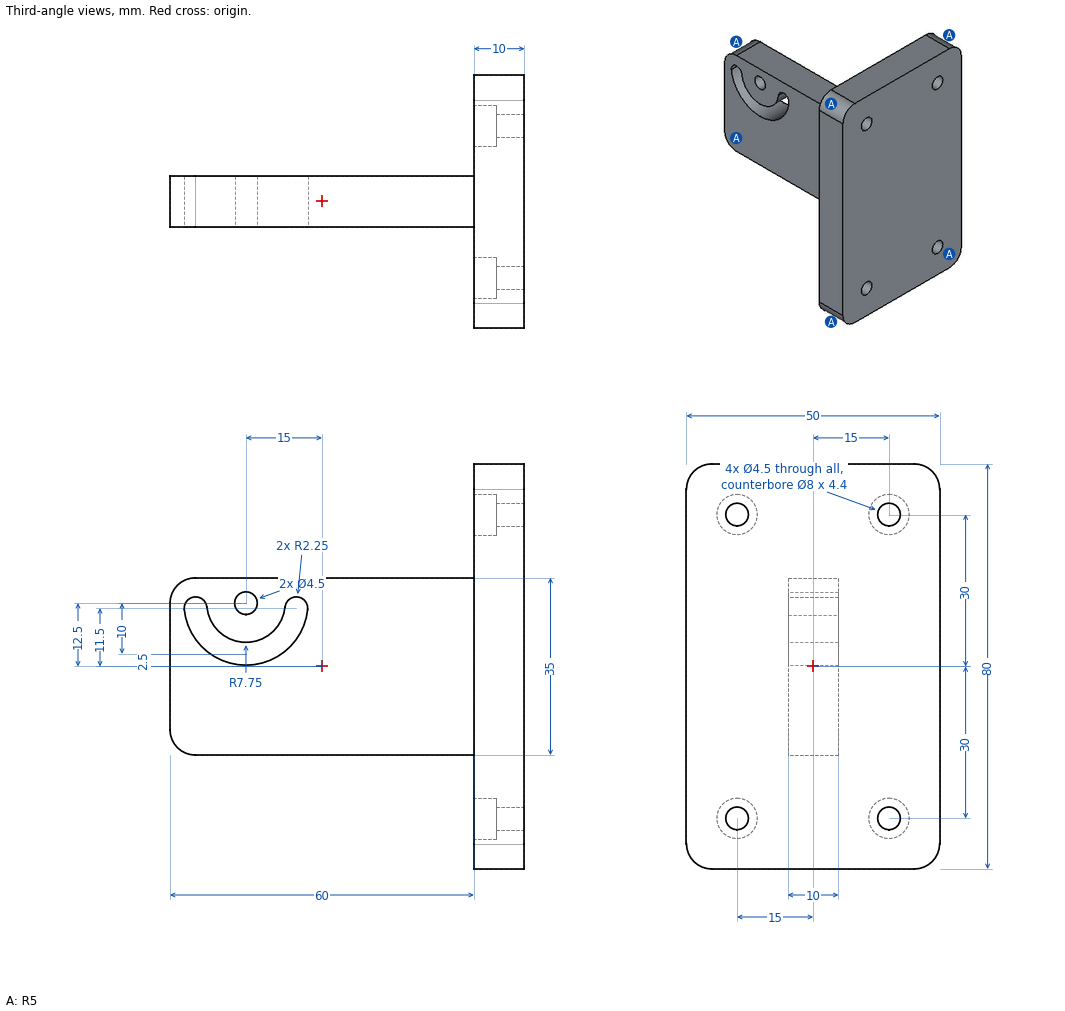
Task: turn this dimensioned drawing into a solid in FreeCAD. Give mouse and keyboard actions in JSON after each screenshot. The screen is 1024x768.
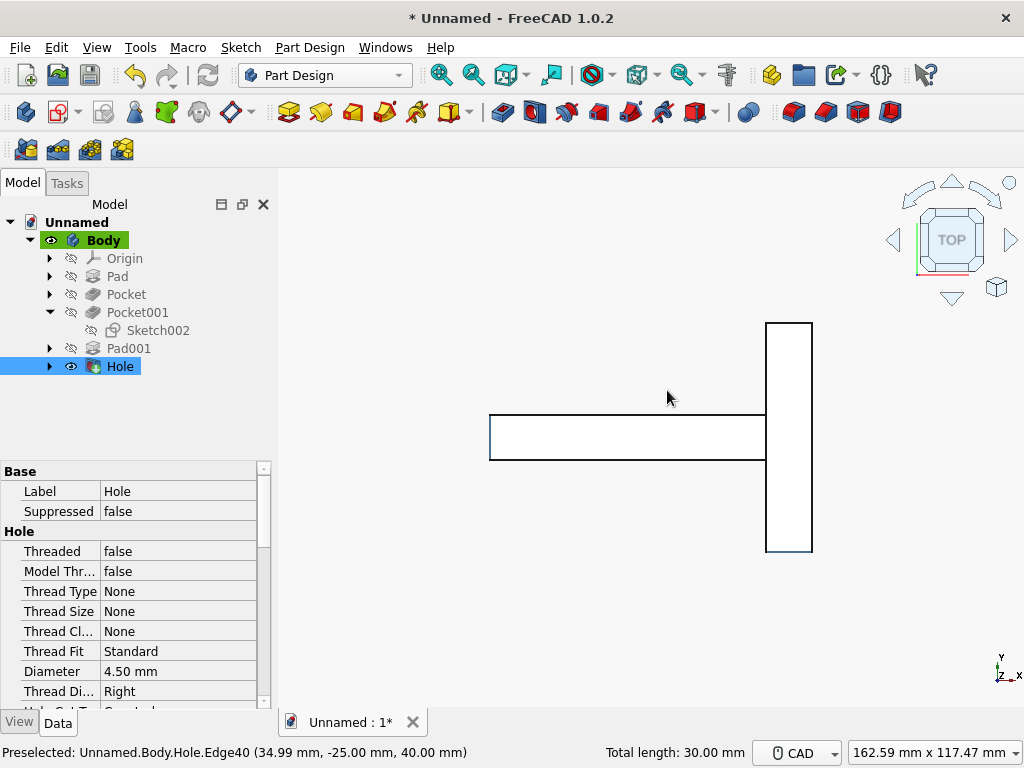
{"action": "left_click", "coordinate": [442, 76]}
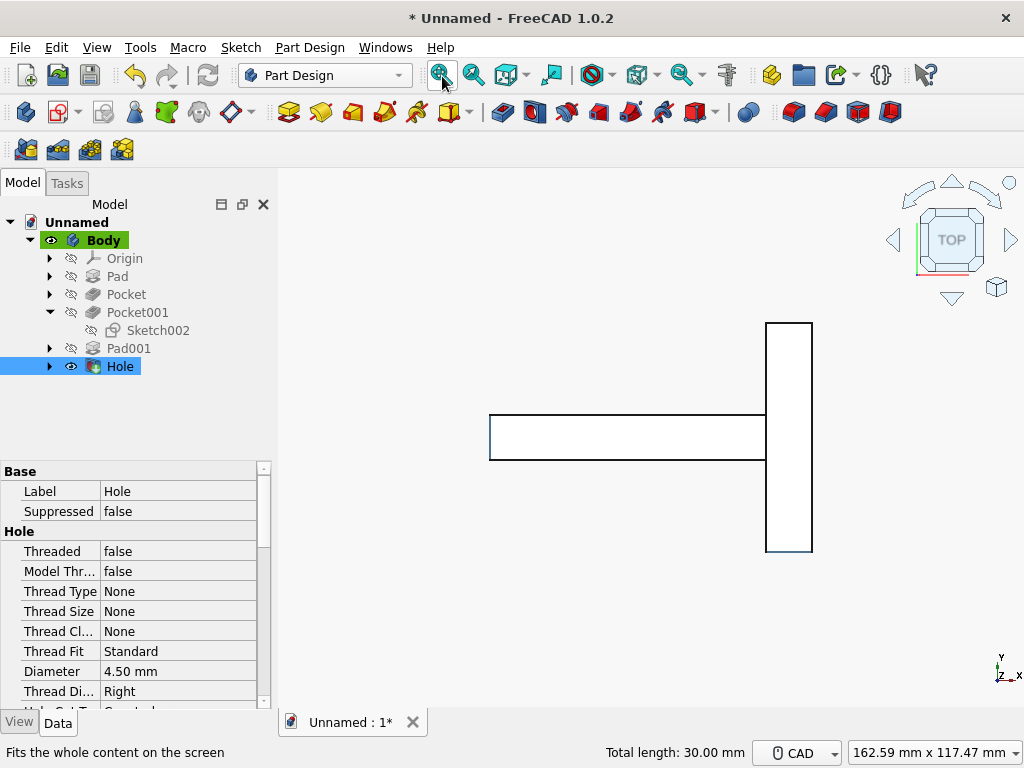
{"action": "left_click", "coordinate": [789, 322], "text": "ctrl"}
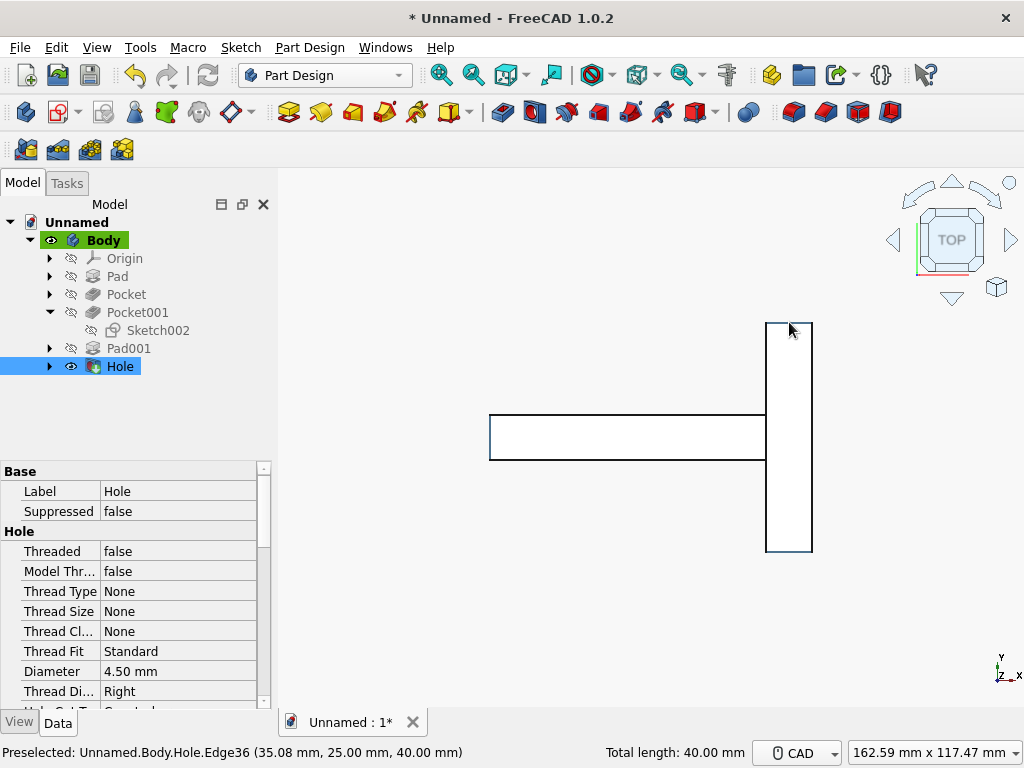
{"action": "key", "text": "1"}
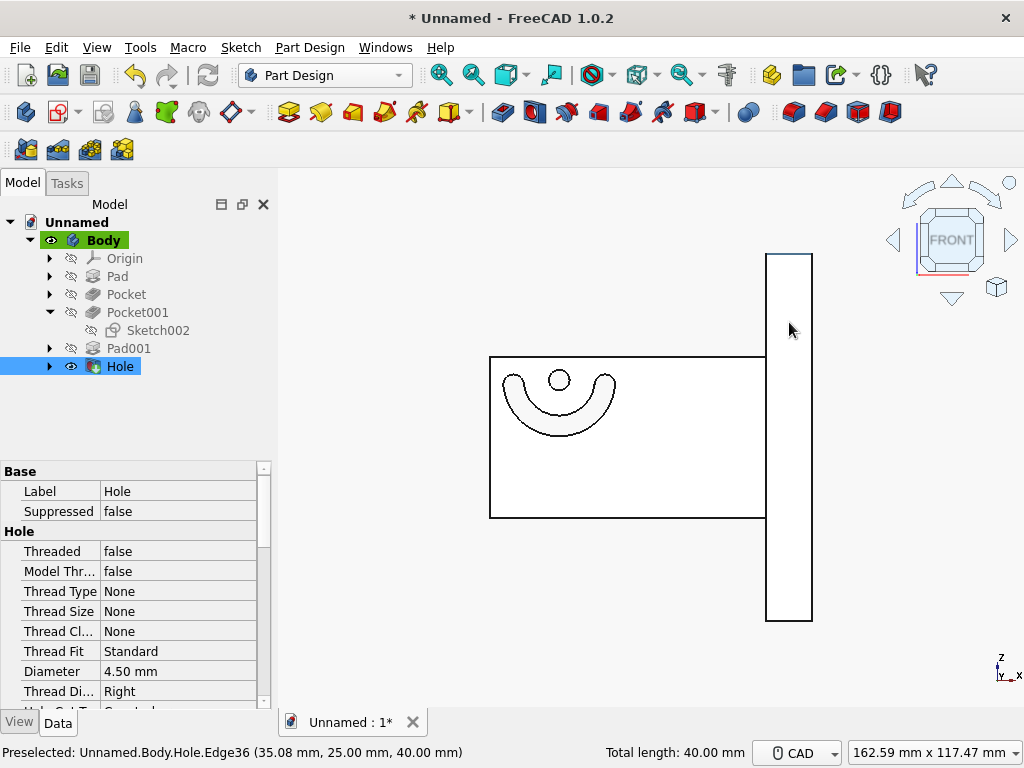
{"action": "key", "text": "3"}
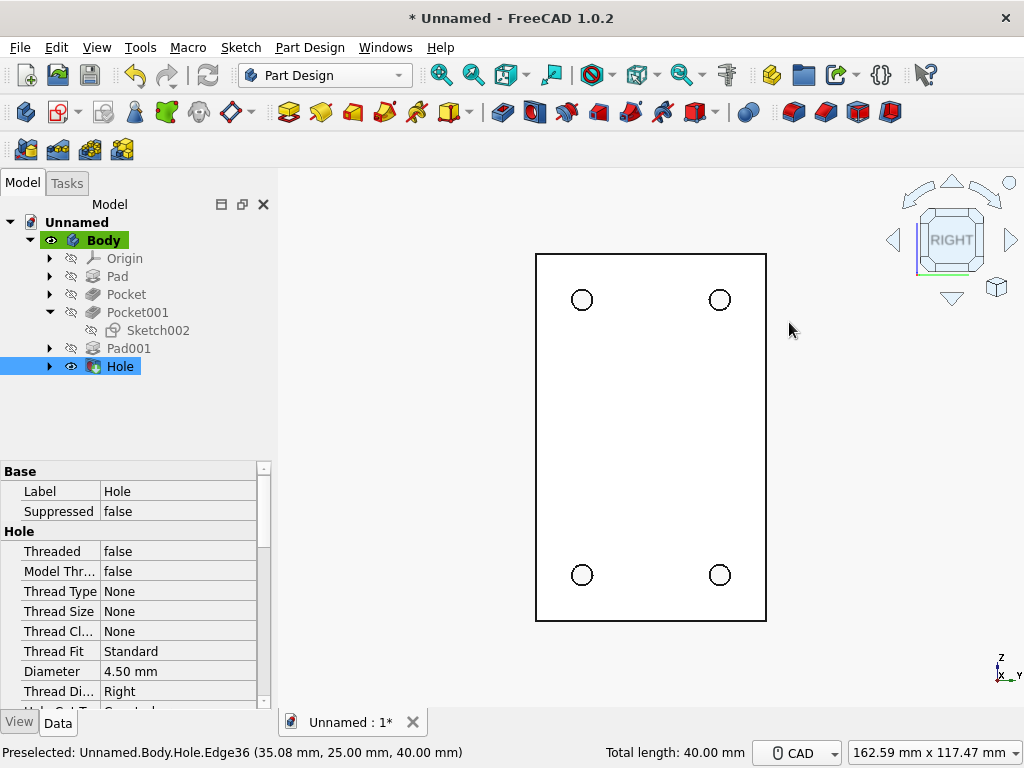
{"action": "key", "text": "5"}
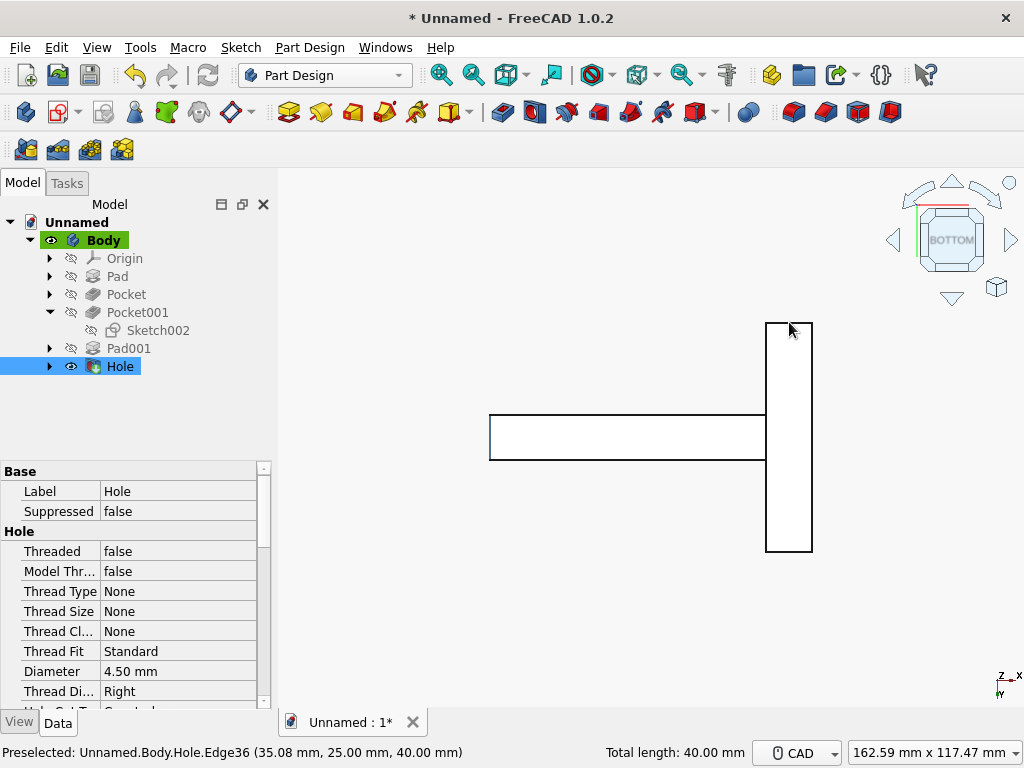
{"action": "left_click", "coordinate": [442, 76]}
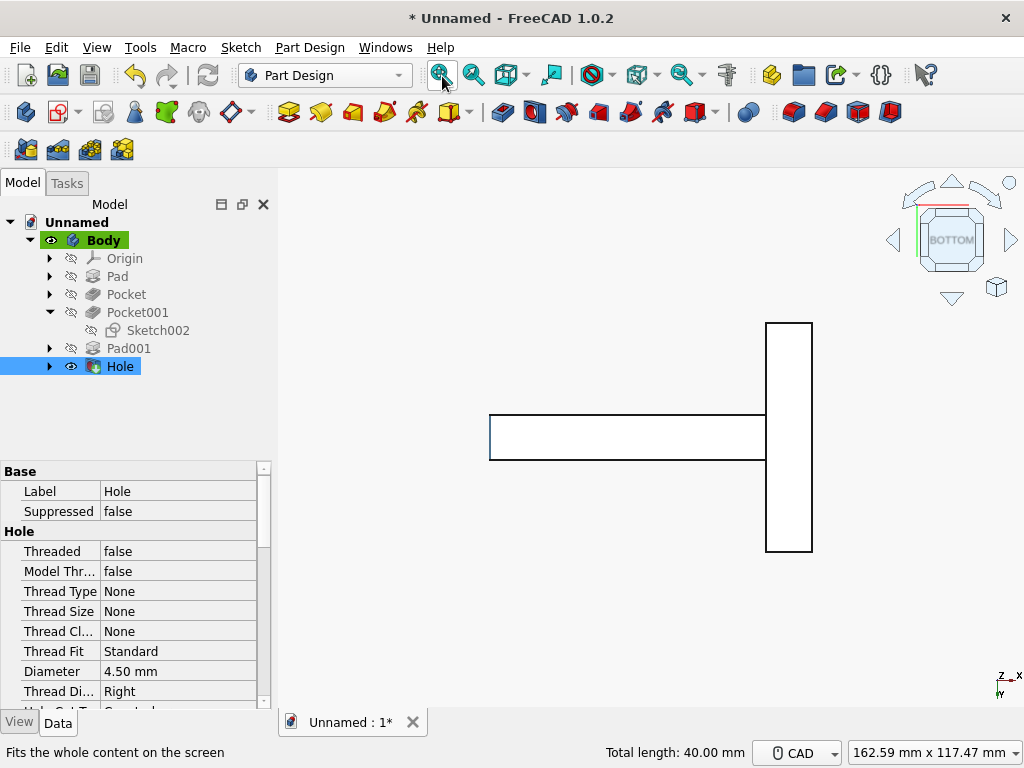
{"action": "left_click", "coordinate": [789, 322], "text": "ctrl"}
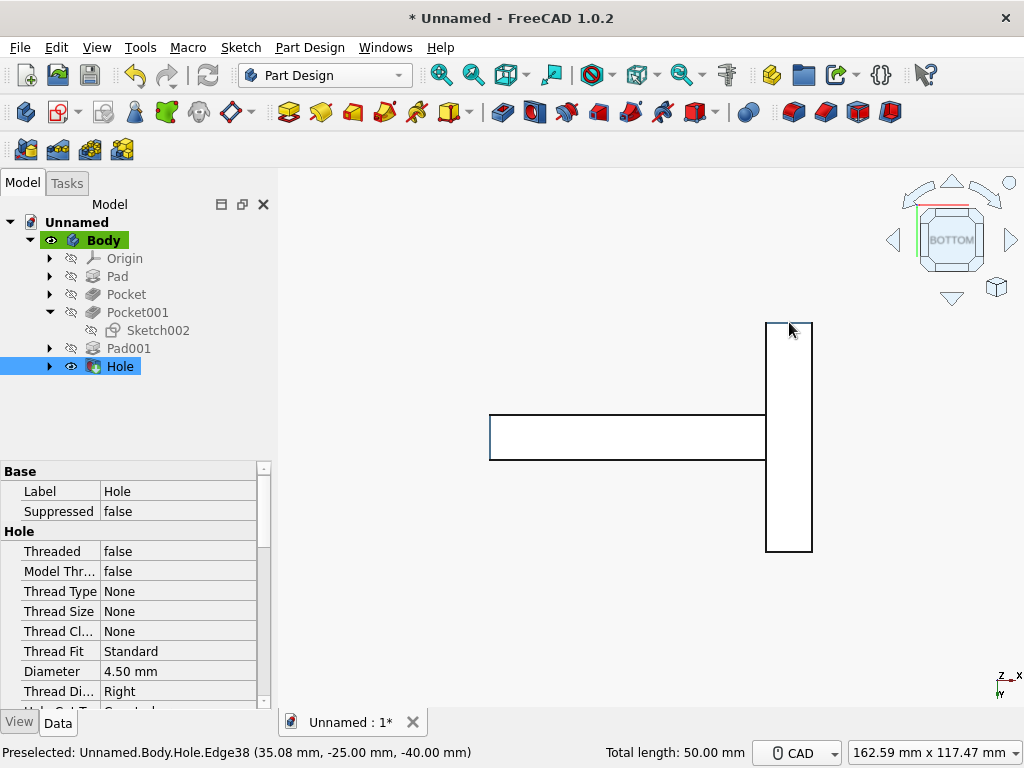
{"action": "key", "text": "4"}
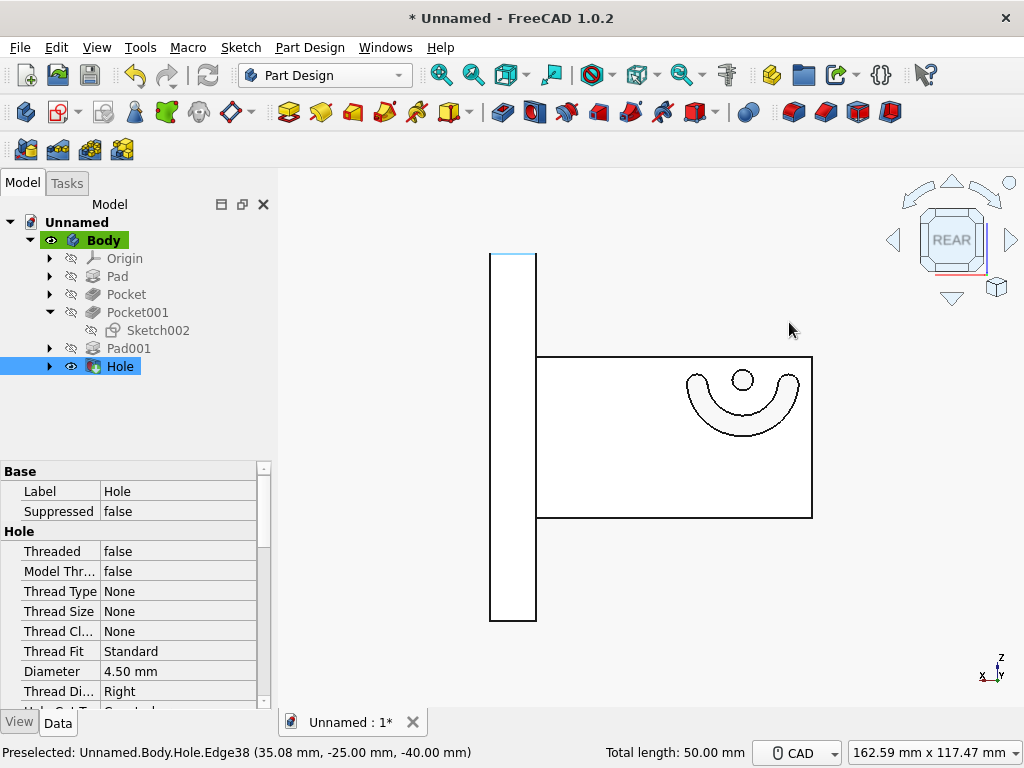
{"action": "left_click", "coordinate": [513, 620], "text": "ctrl"}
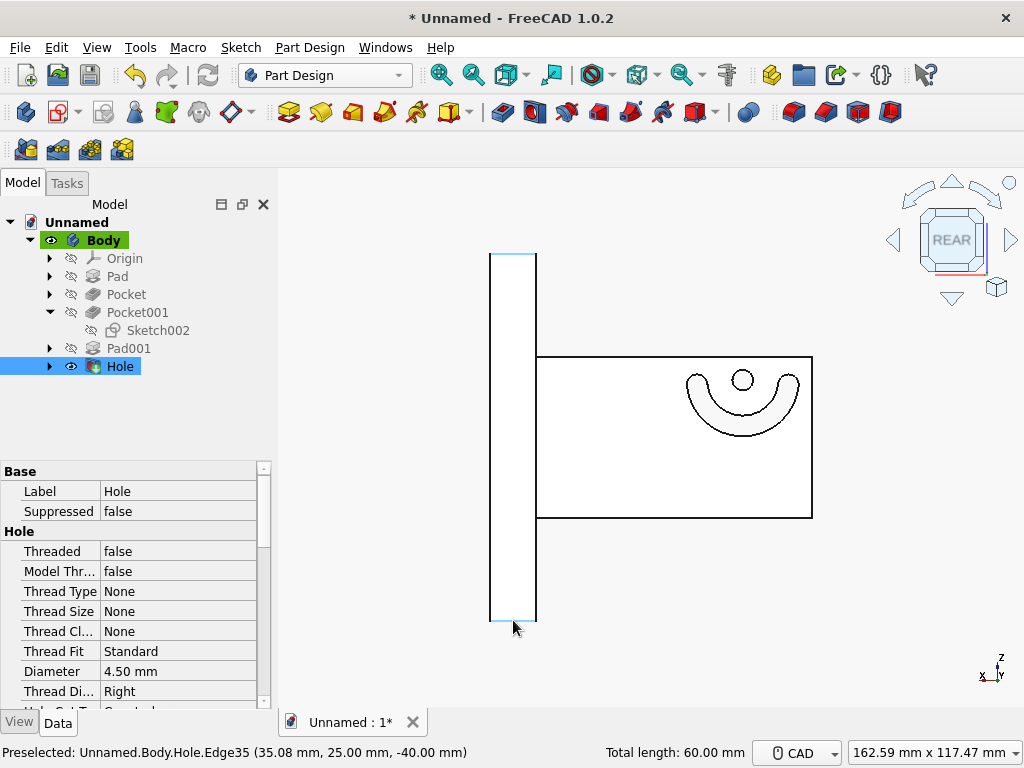
{"action": "left_click", "coordinate": [794, 112]}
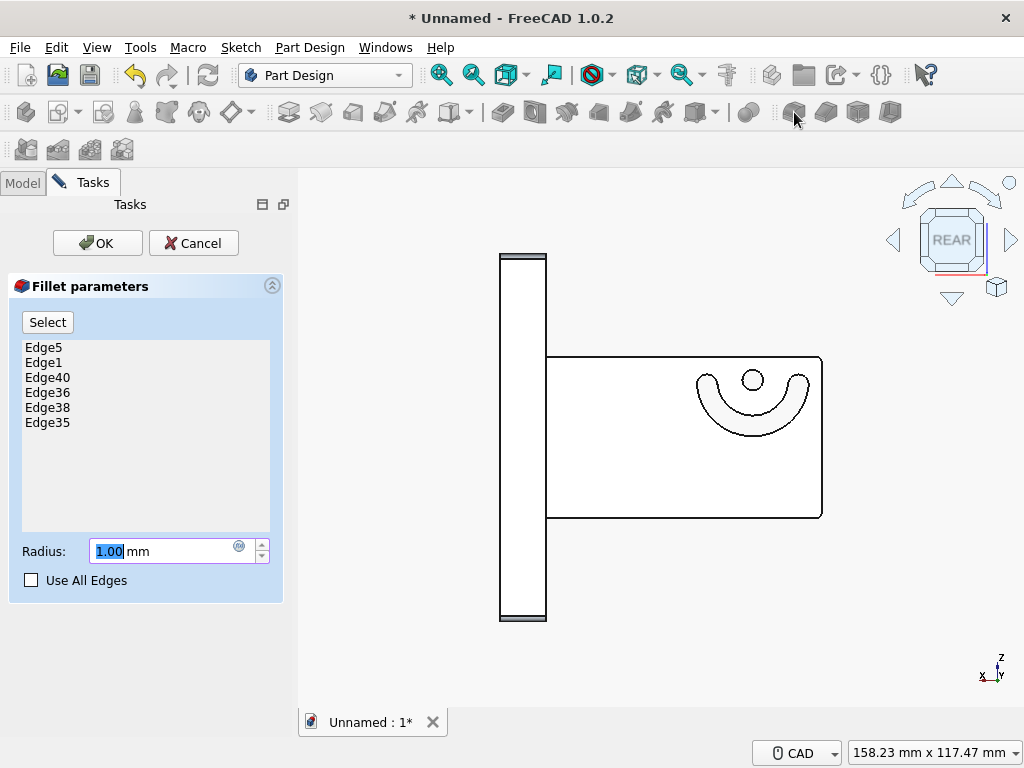
{"action": "type", "text": "5"}
{"action": "key", "text": "Tab"}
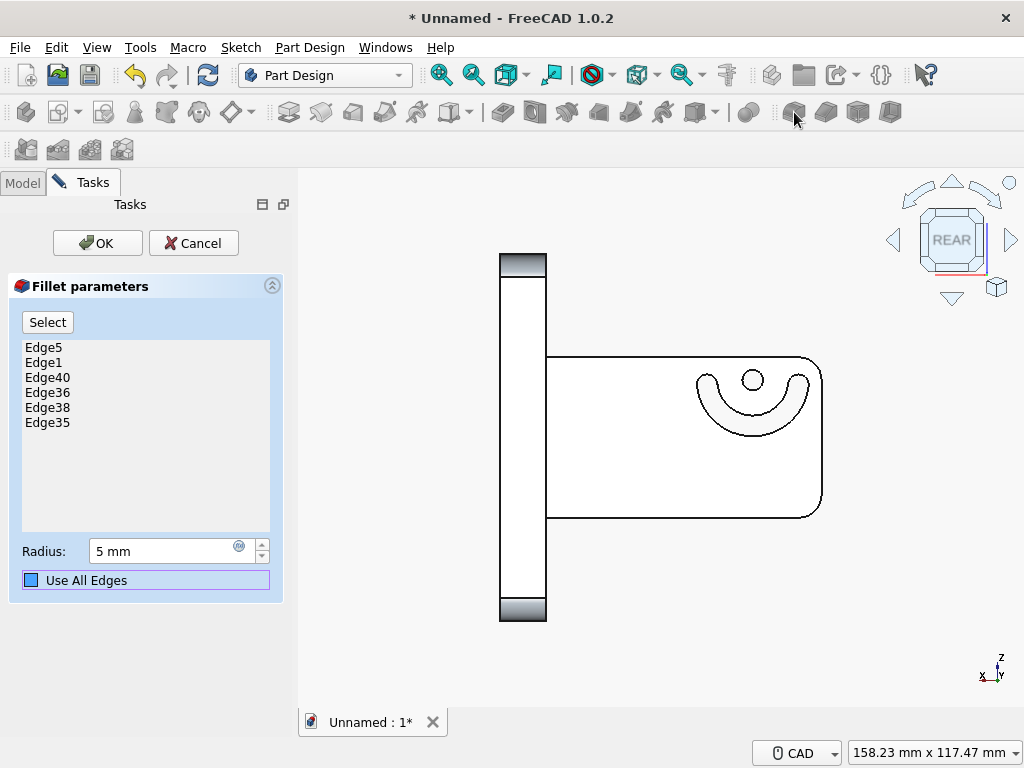
{"action": "left_click", "coordinate": [98, 243]}